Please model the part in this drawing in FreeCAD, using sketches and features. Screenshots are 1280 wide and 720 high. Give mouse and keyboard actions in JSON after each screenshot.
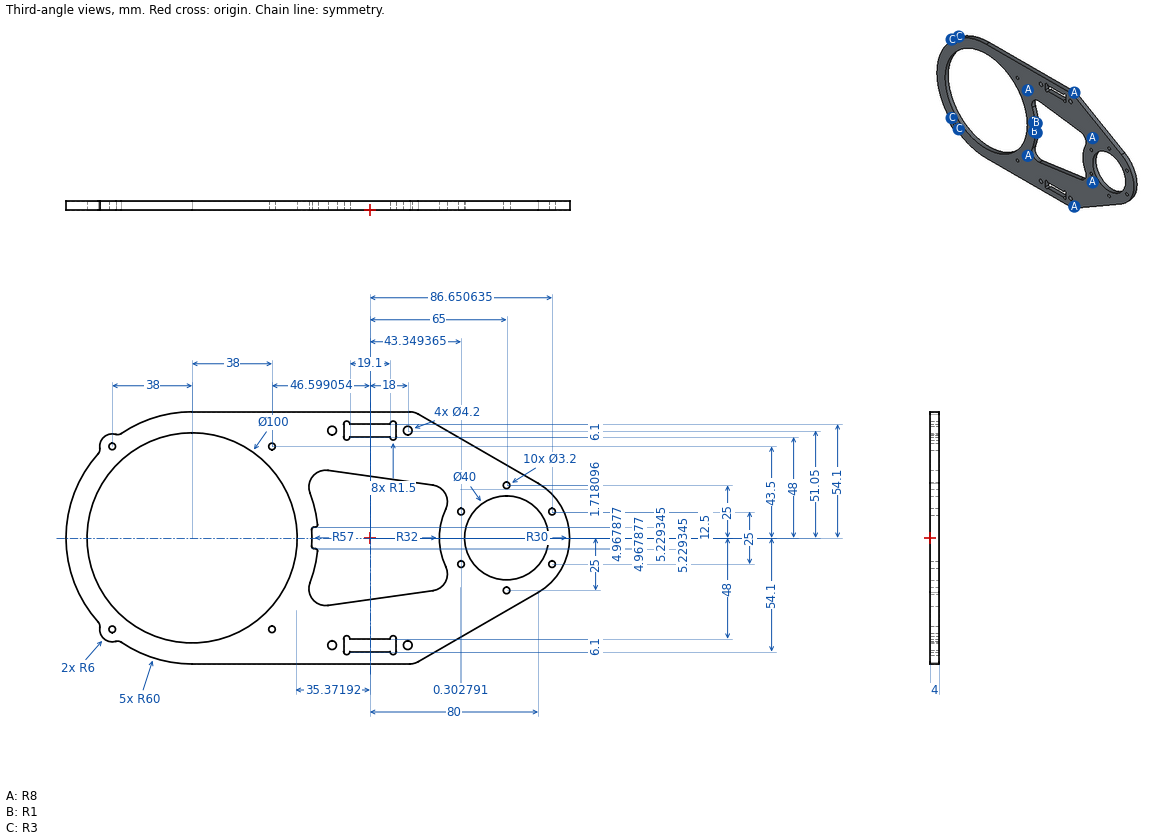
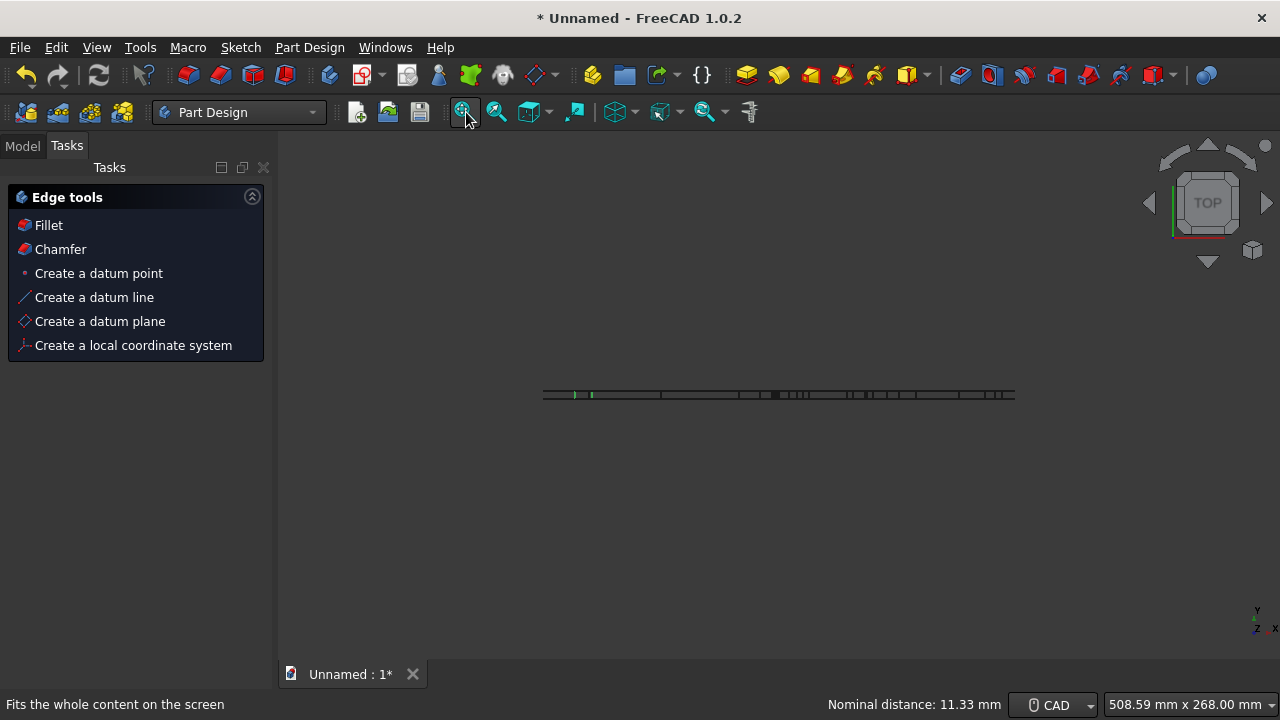
{"action": "key", "text": "1"}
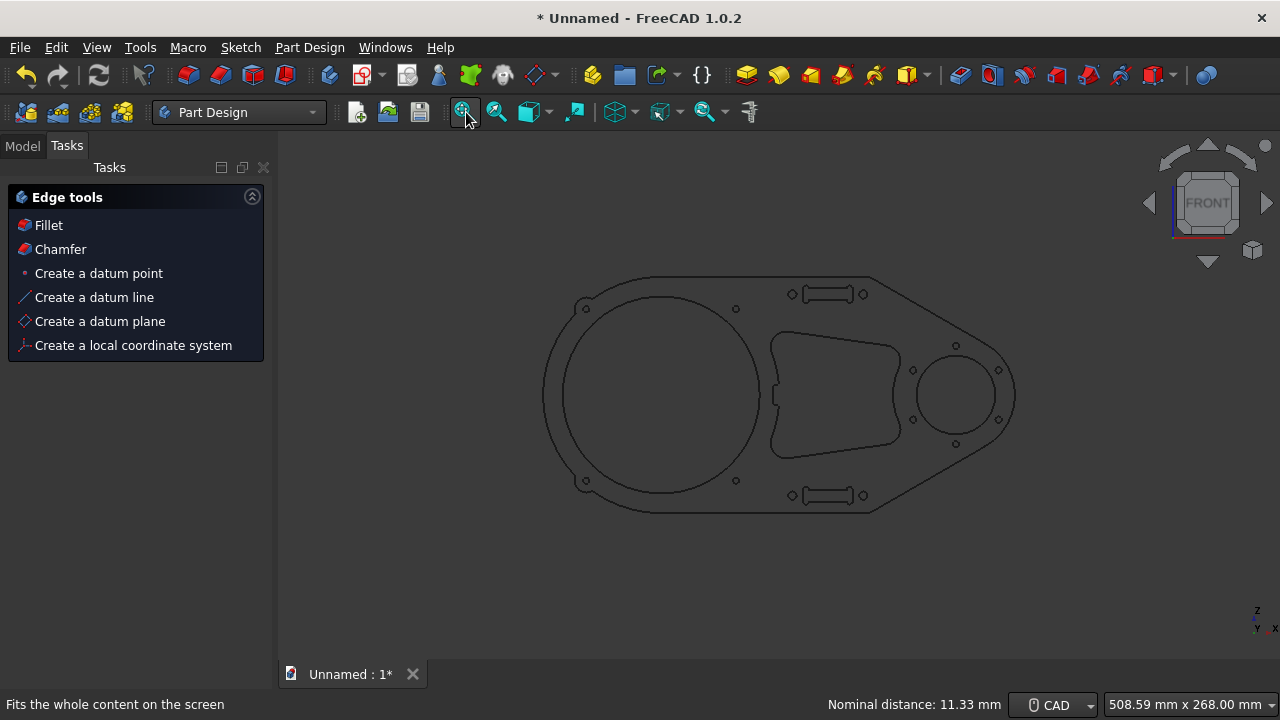
{"action": "scroll", "coordinate": [575, 475], "scroll_direction": "up", "scroll_amount": 9}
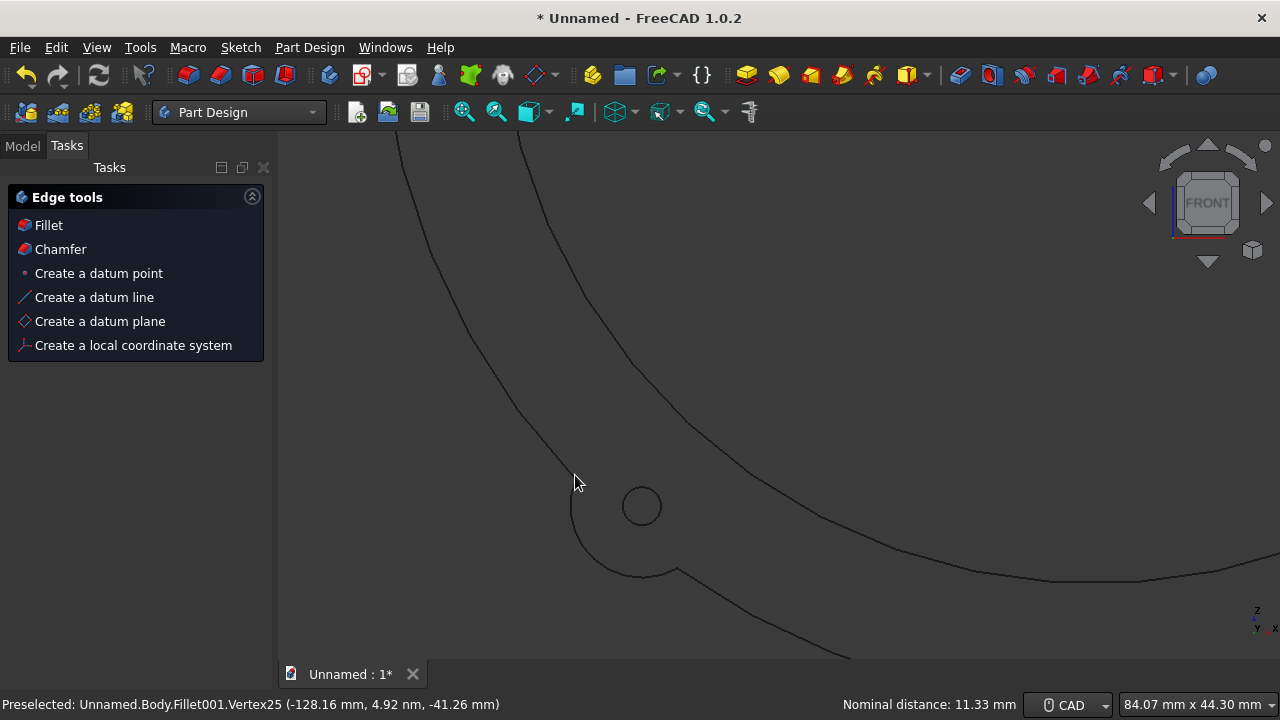
{"action": "left_click", "coordinate": [466, 112]}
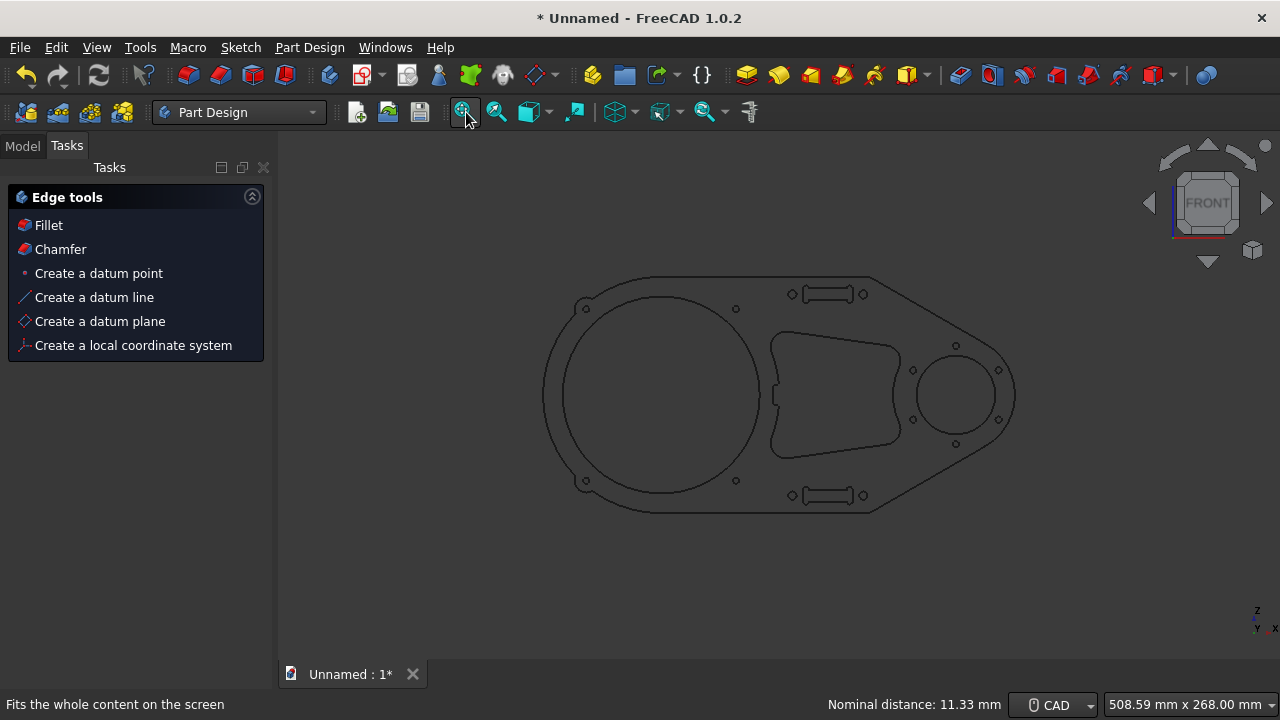
{"action": "key", "text": "3"}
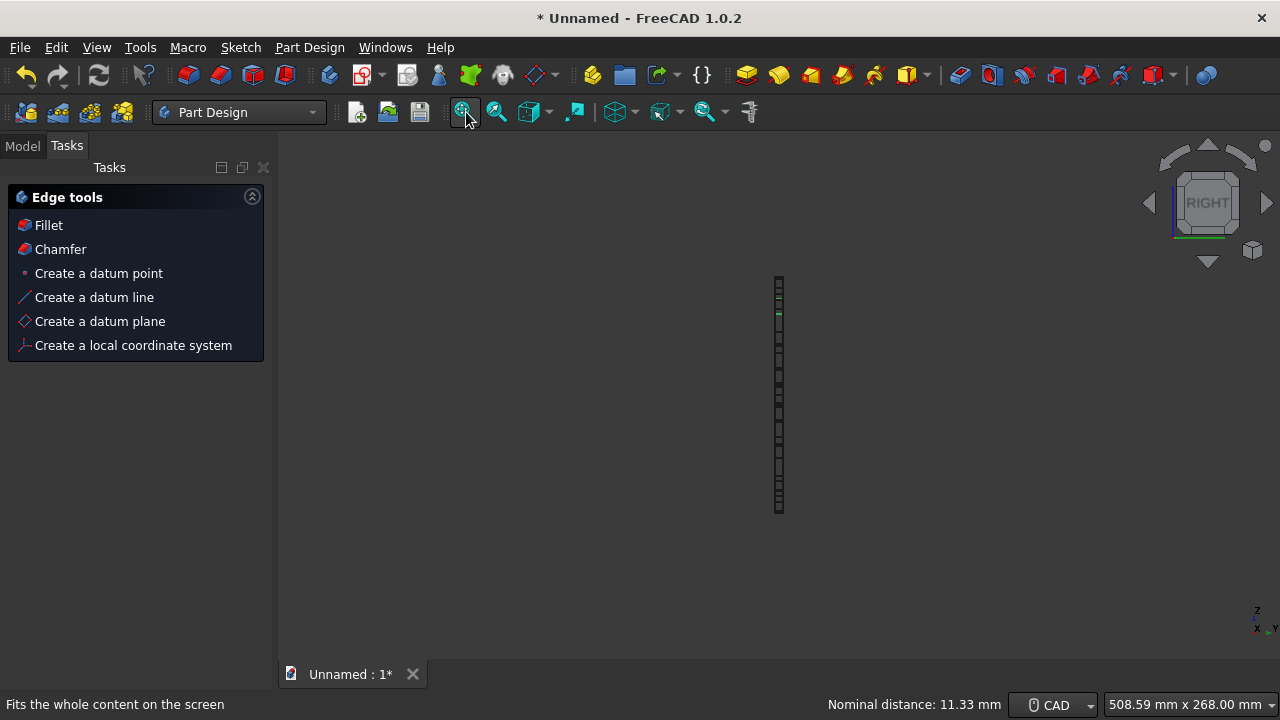
{"action": "left_click", "coordinate": [466, 112]}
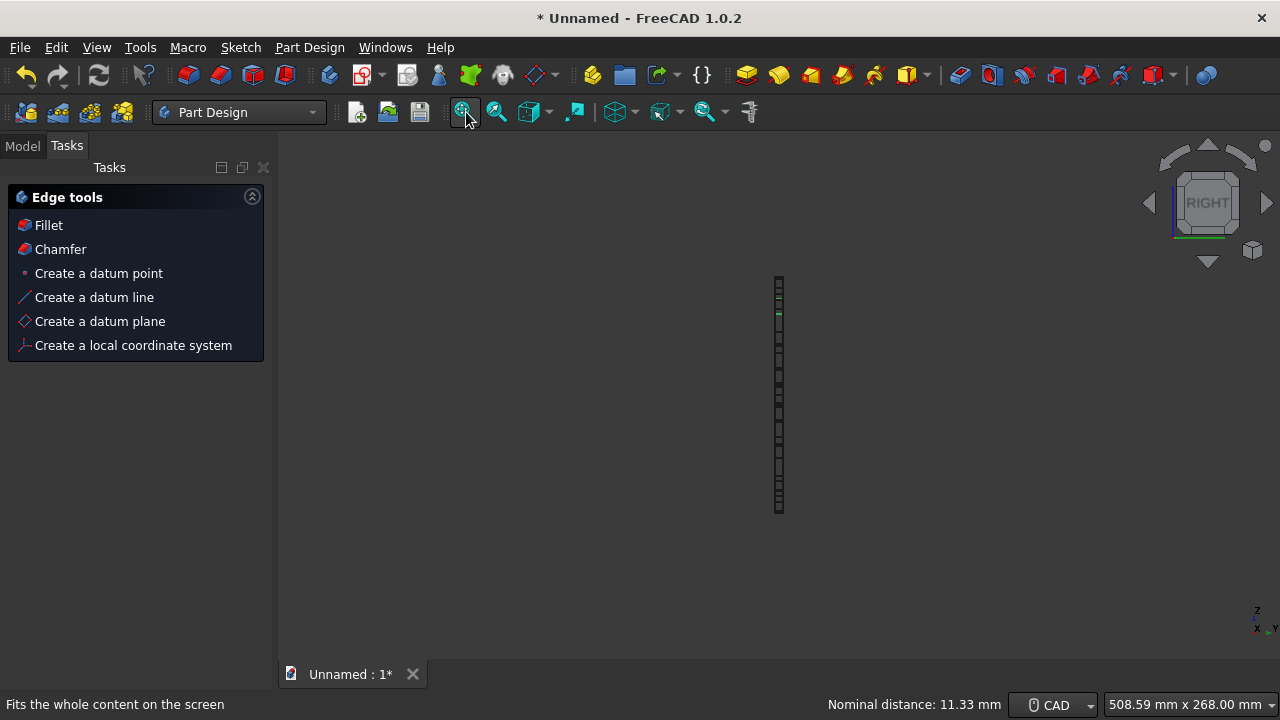
{"action": "scroll", "coordinate": [779, 475], "scroll_direction": "up", "scroll_amount": 9}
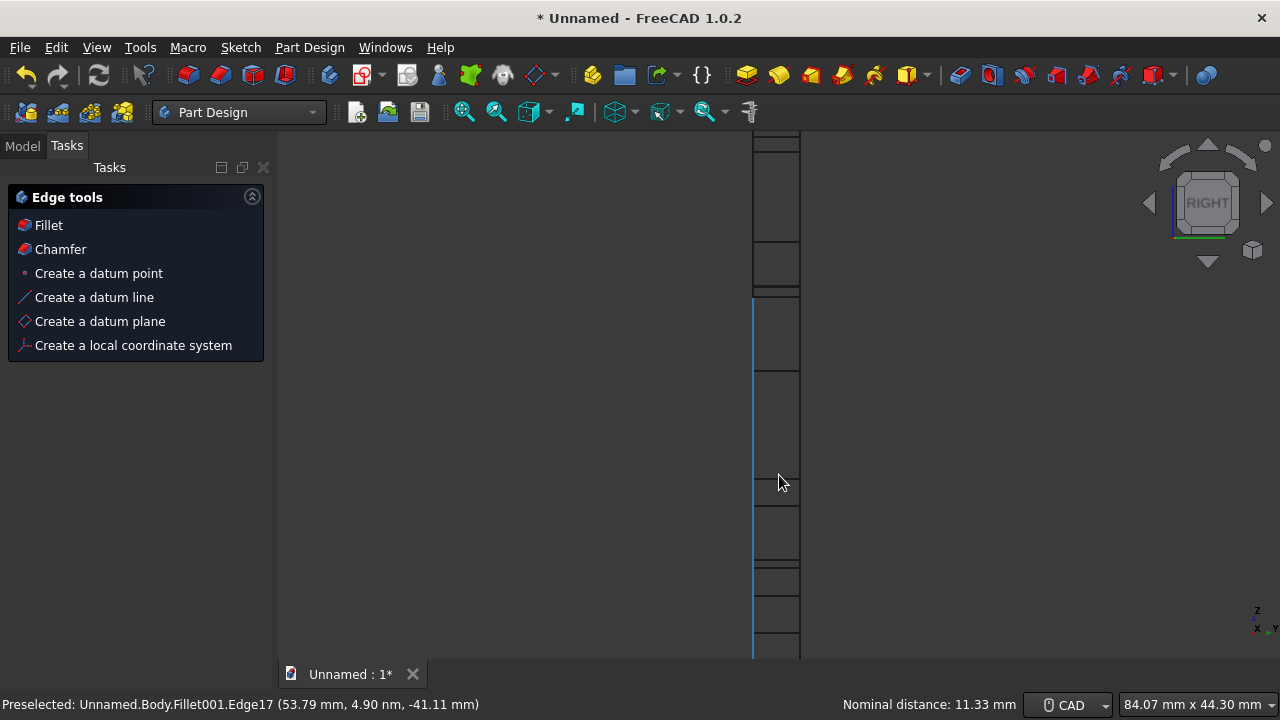
{"action": "left_click", "coordinate": [776, 478], "text": "ctrl"}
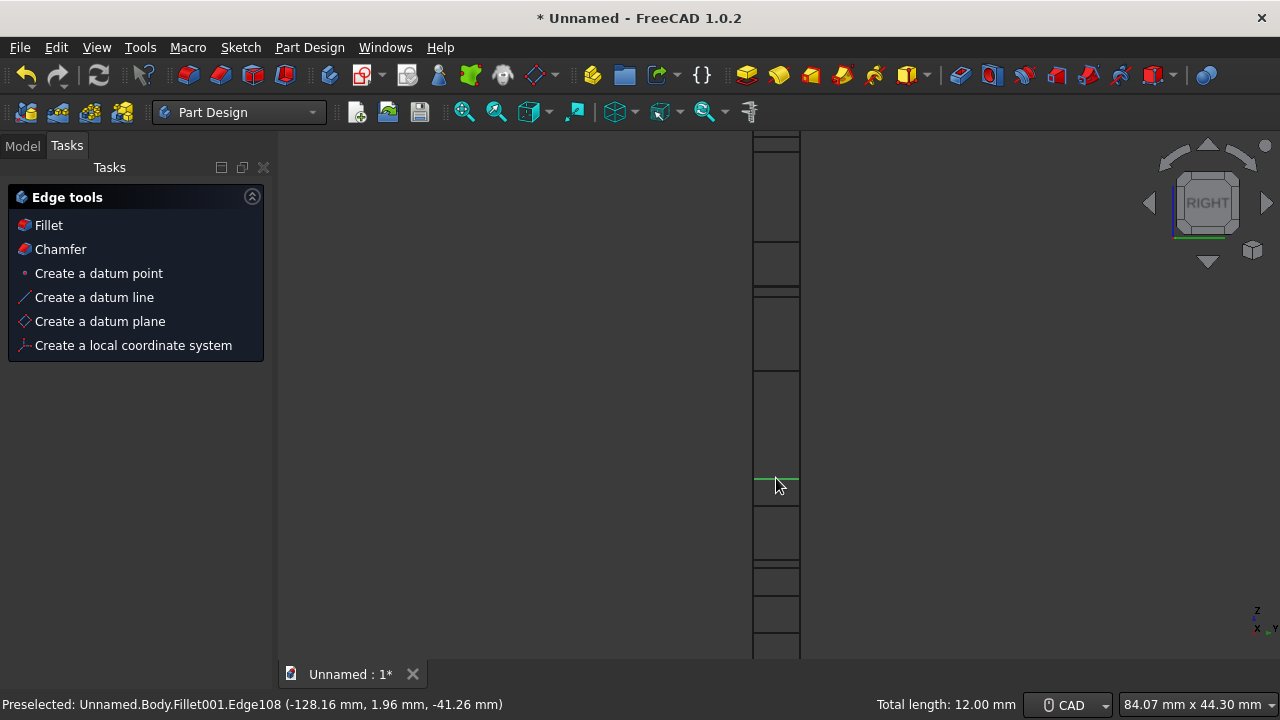
{"action": "left_click", "coordinate": [776, 567], "text": "ctrl"}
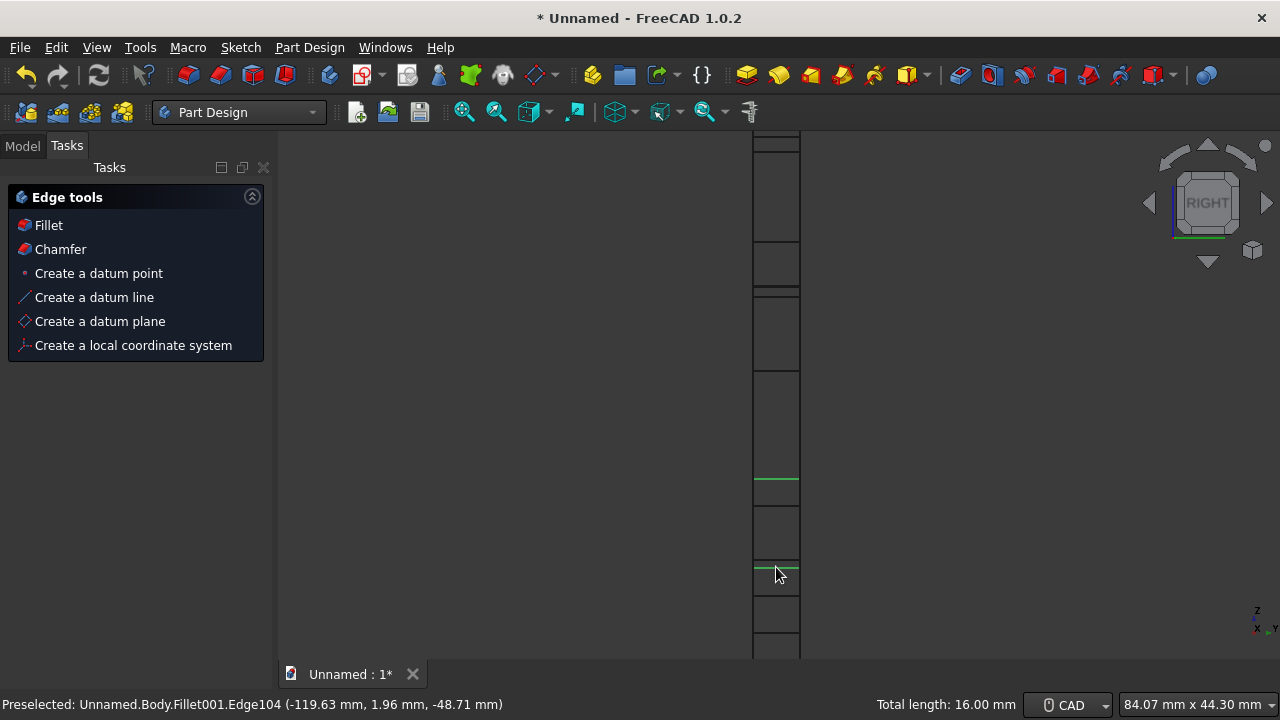
{"action": "key", "text": "v 1"}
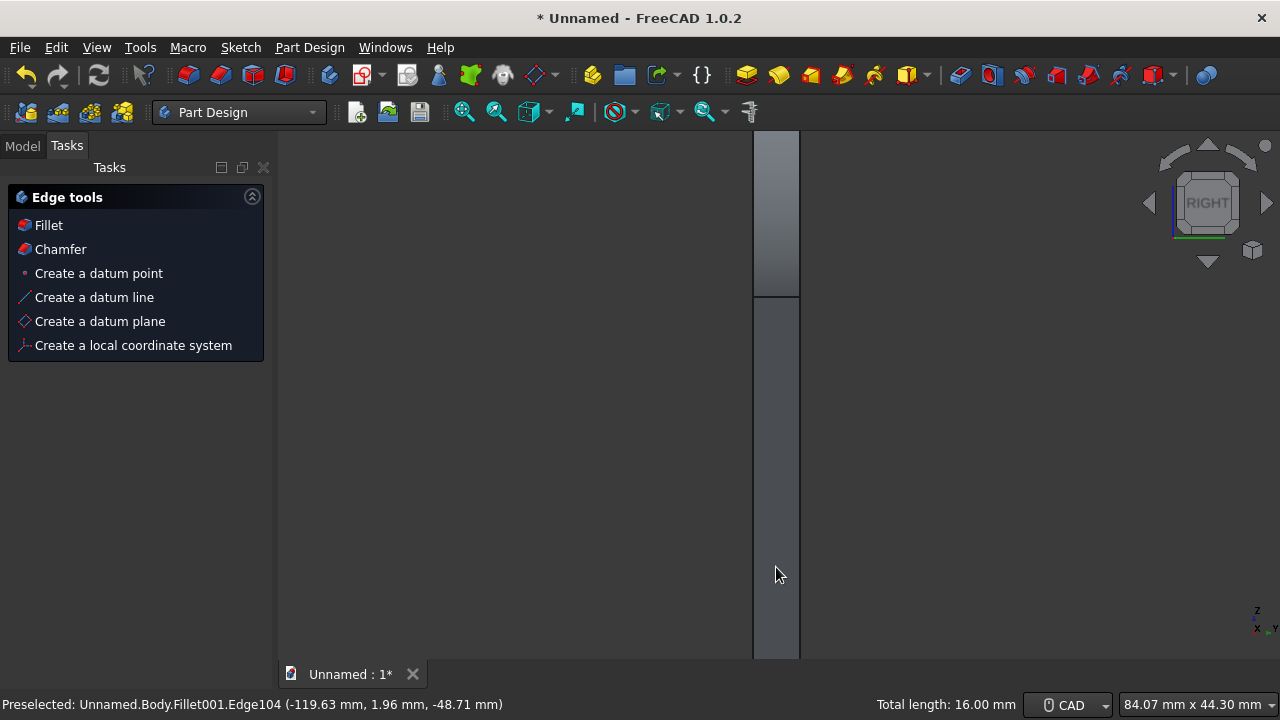
{"action": "left_click", "coordinate": [190, 76]}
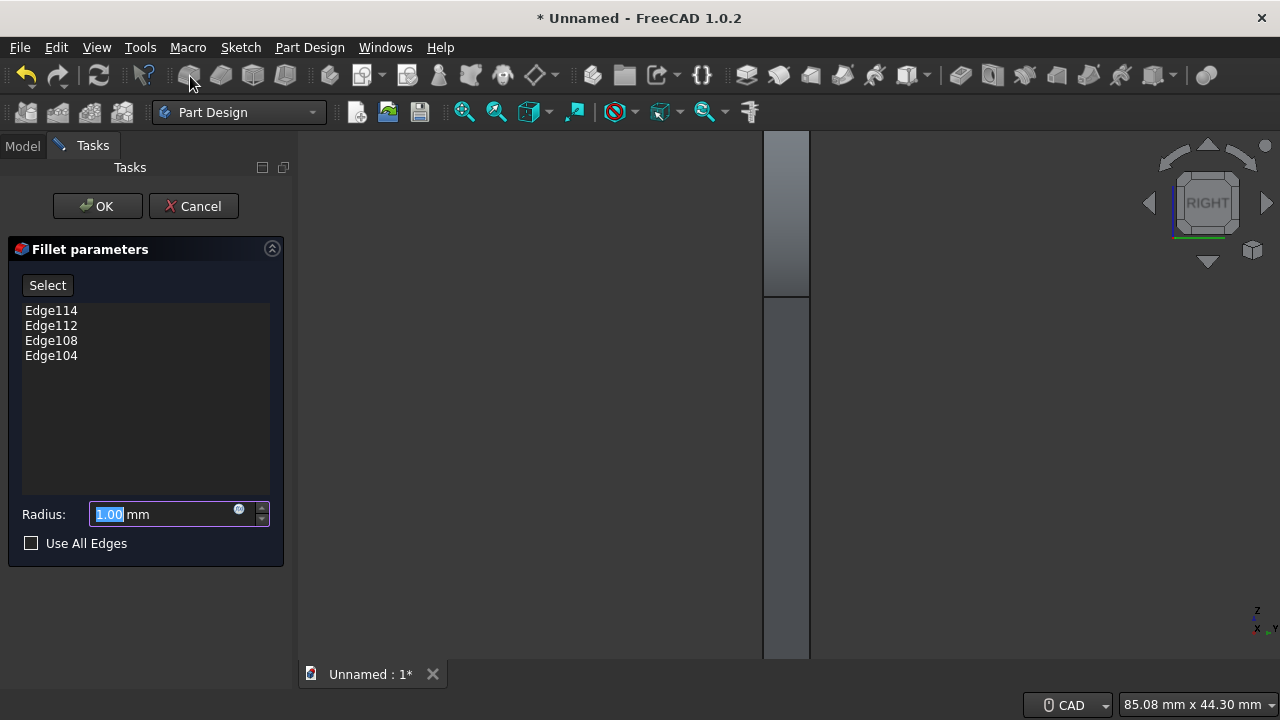
{"action": "type", "text": "3"}
{"action": "key", "text": "Tab"}